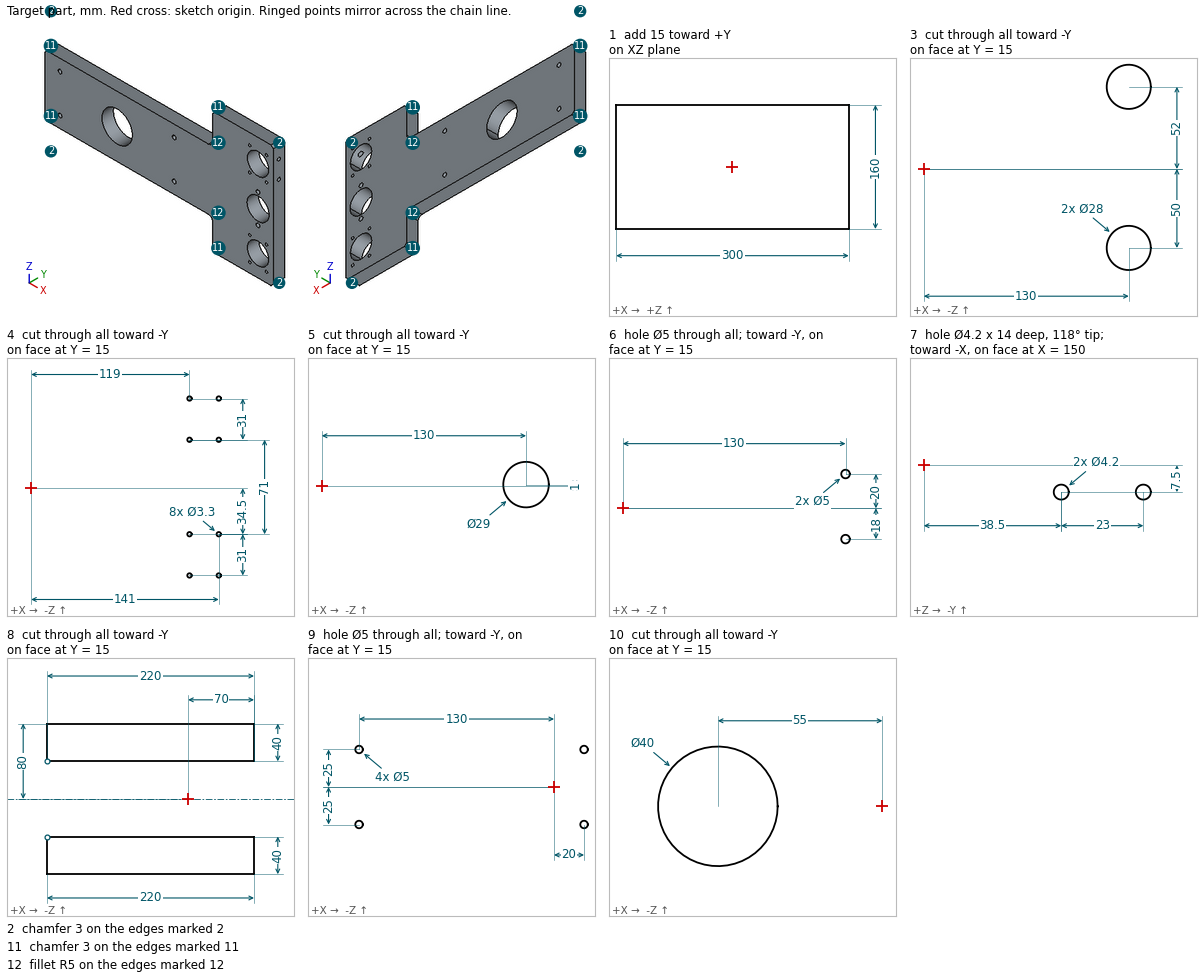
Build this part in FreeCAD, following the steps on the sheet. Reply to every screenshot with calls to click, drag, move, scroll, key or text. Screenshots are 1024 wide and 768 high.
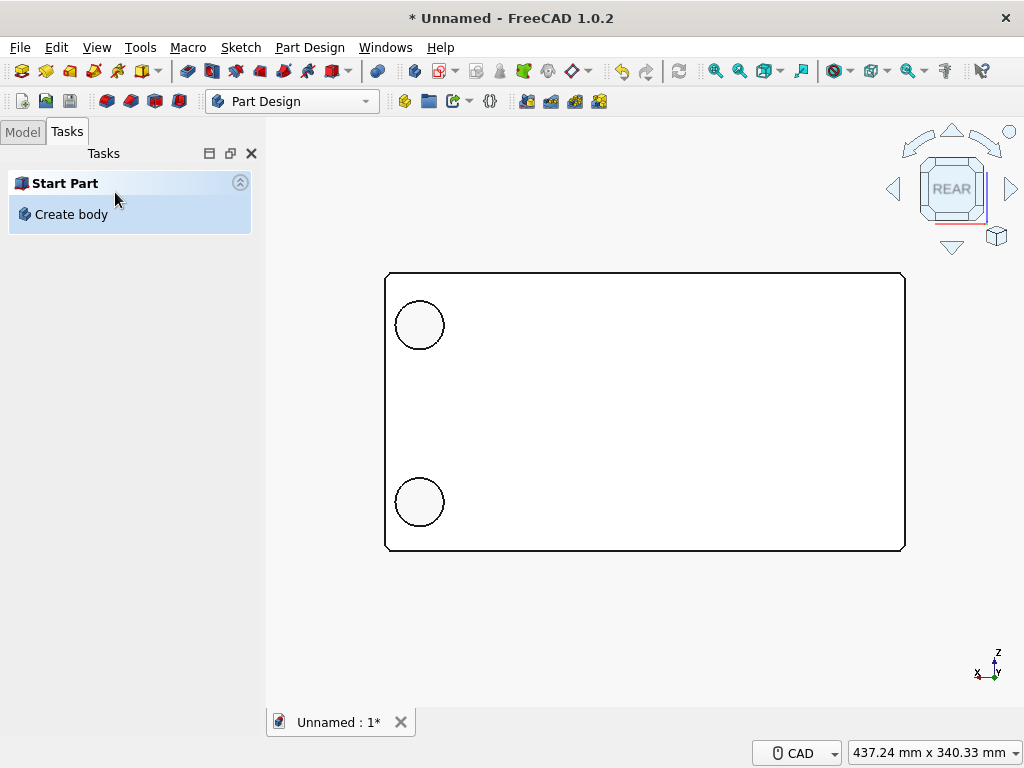
click(571, 411)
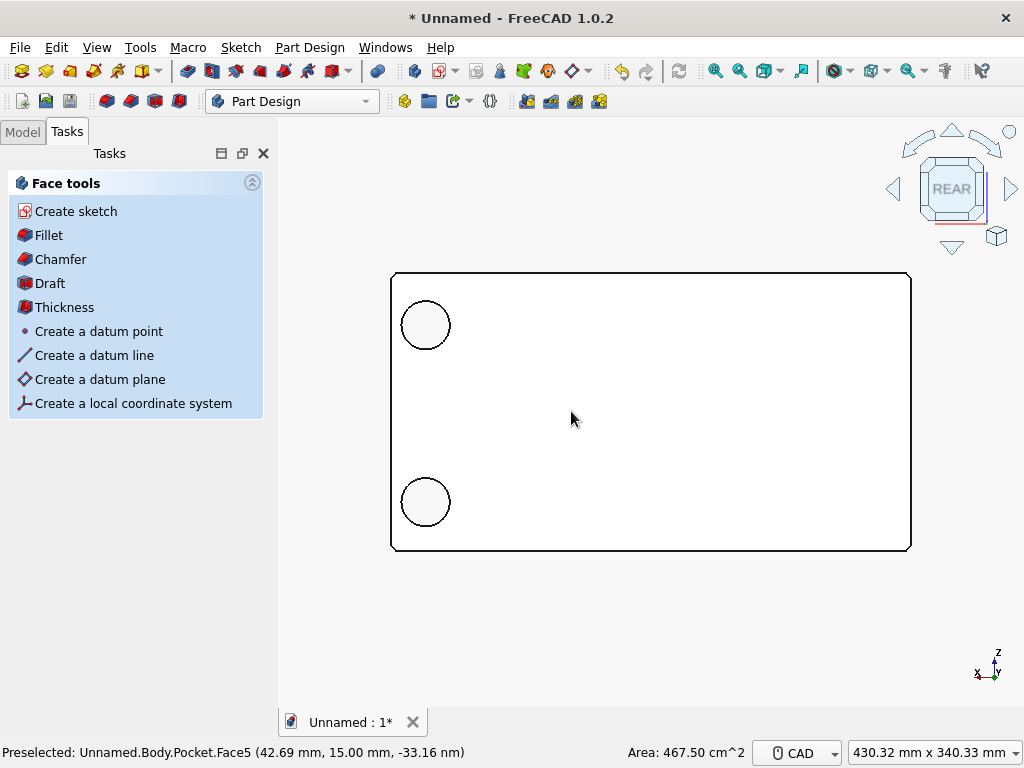
click(440, 72)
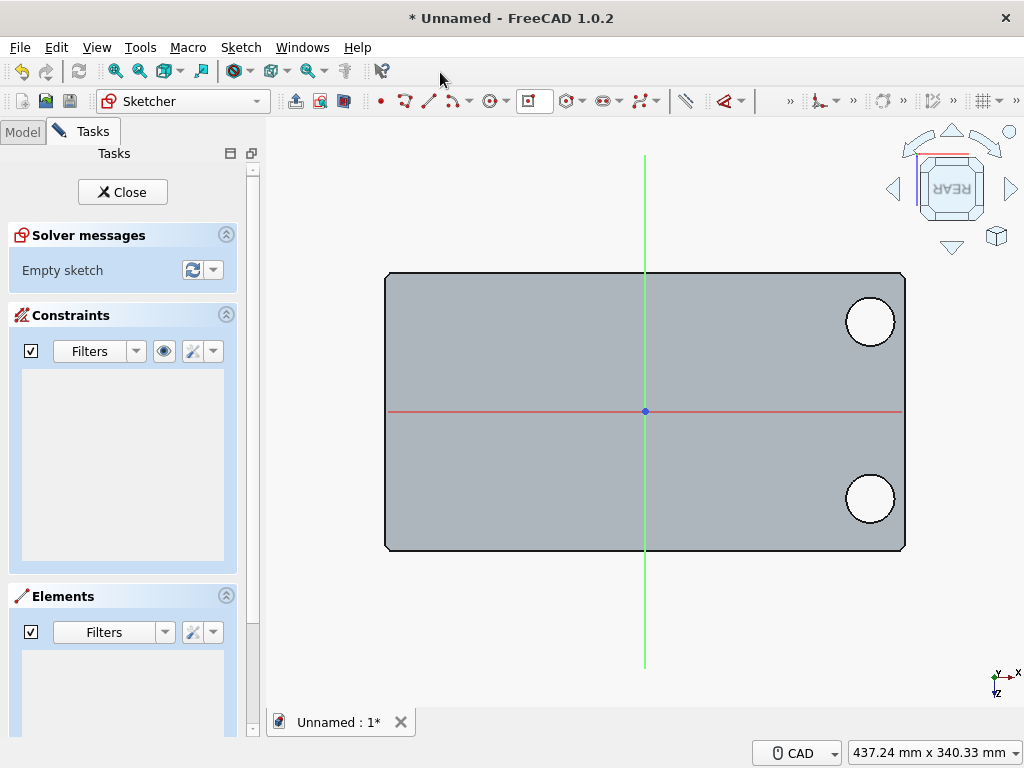
scroll(294, 420, down, 1)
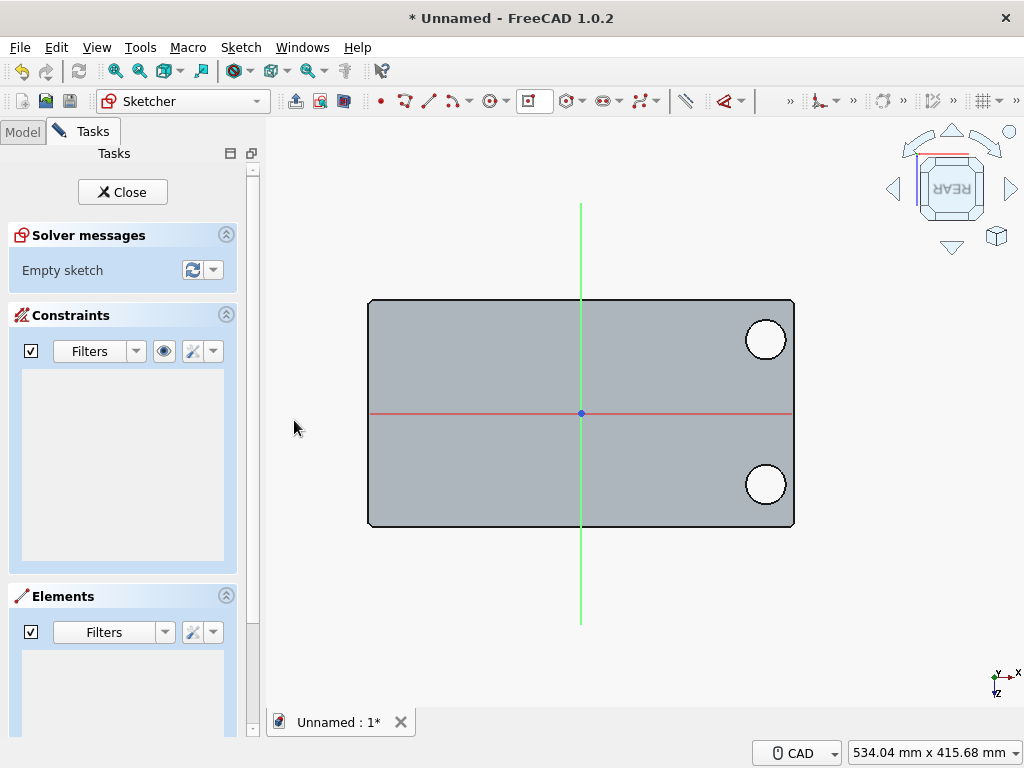
scroll(812, 412, up, 3)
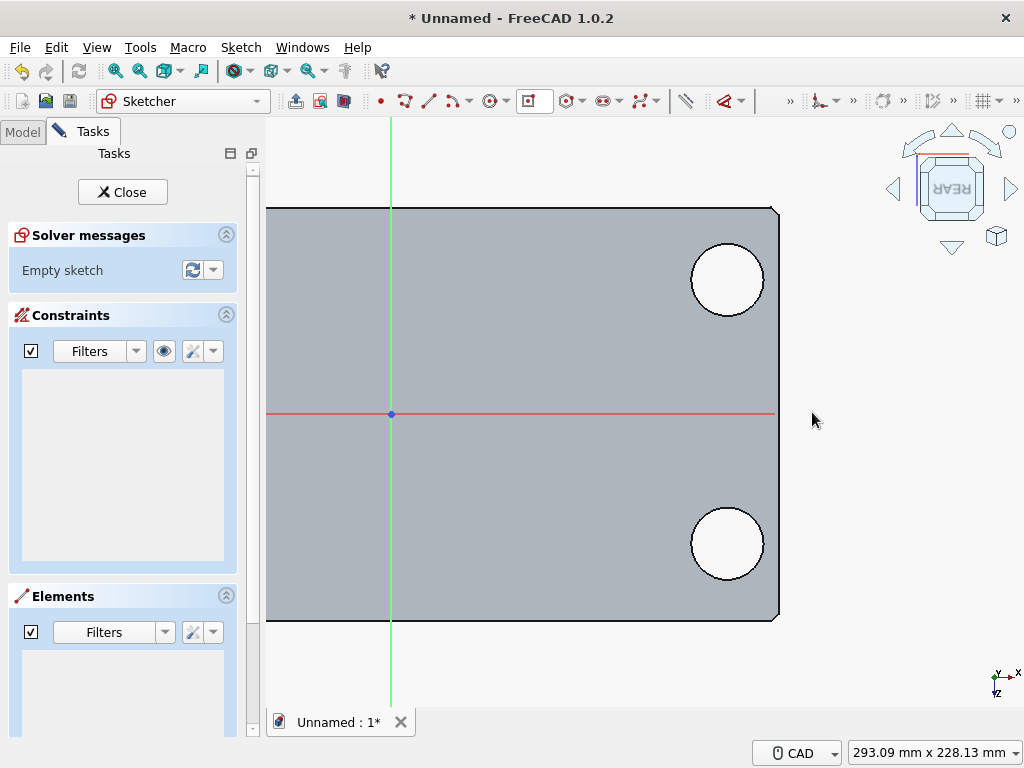
click(490, 102)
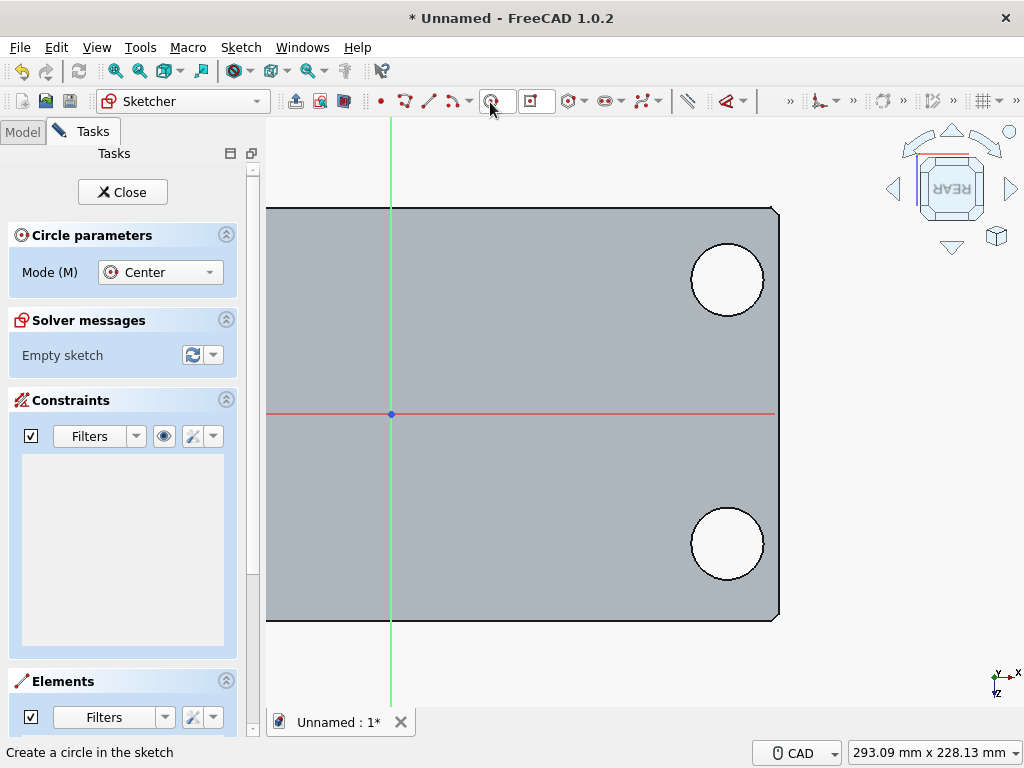
scroll(756, 504, up, 9)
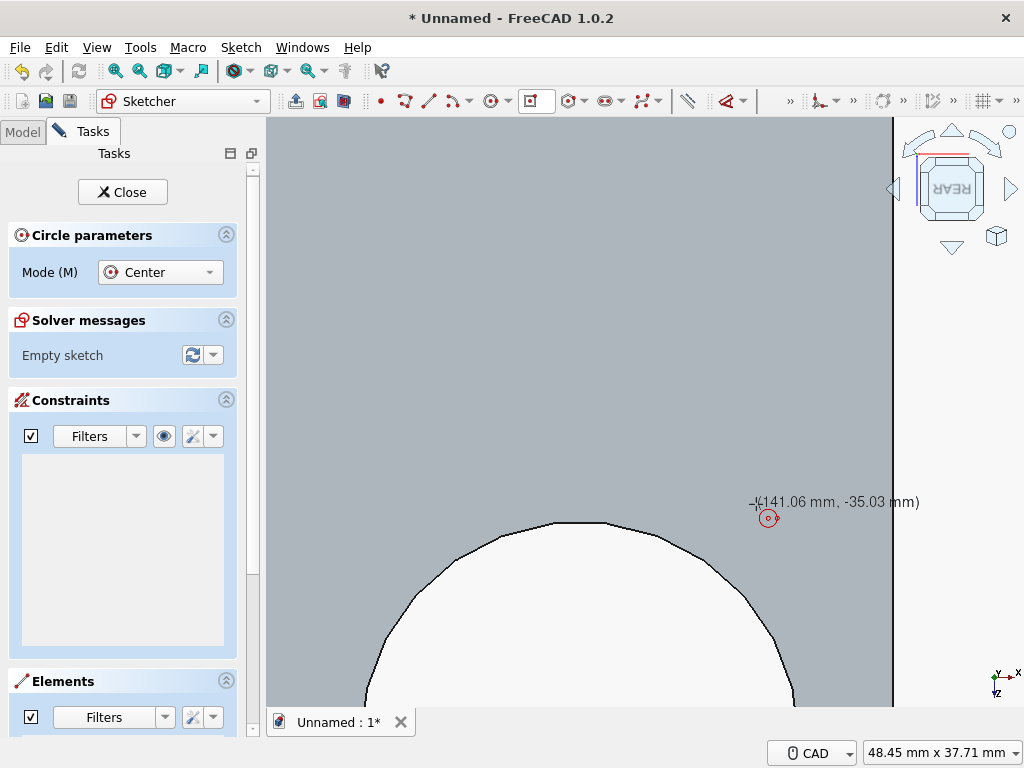
scroll(758, 505, down, 9)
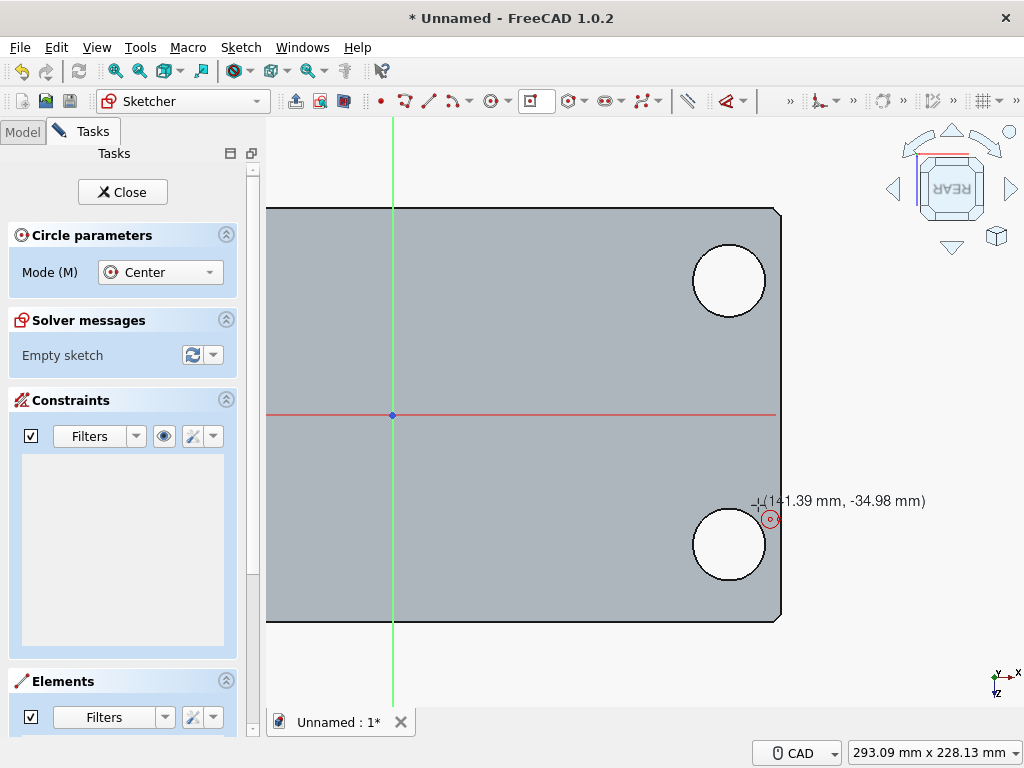
click(758, 504)
move(761, 501)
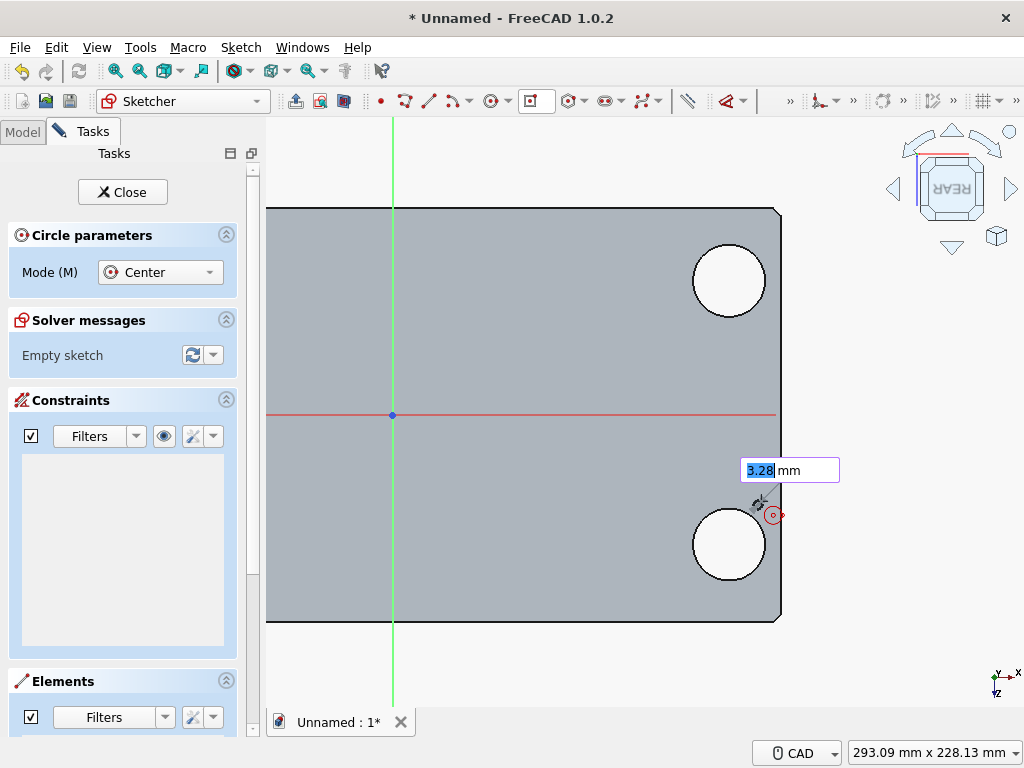
text(3.3)
key(Return)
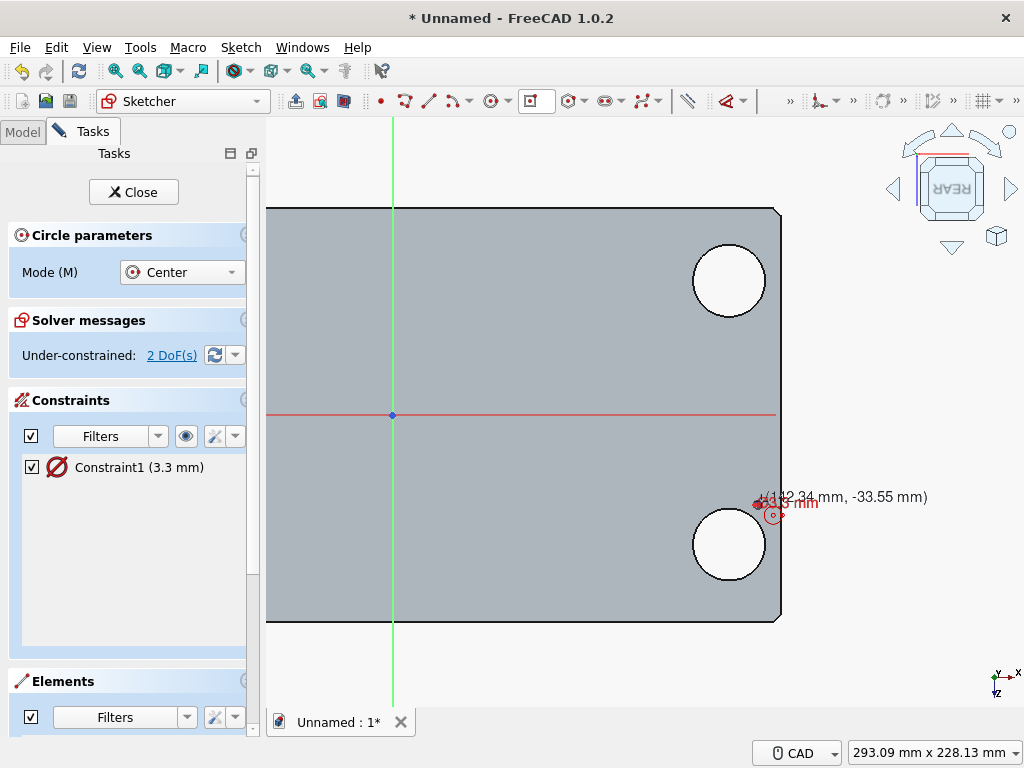
scroll(701, 241, up, 9)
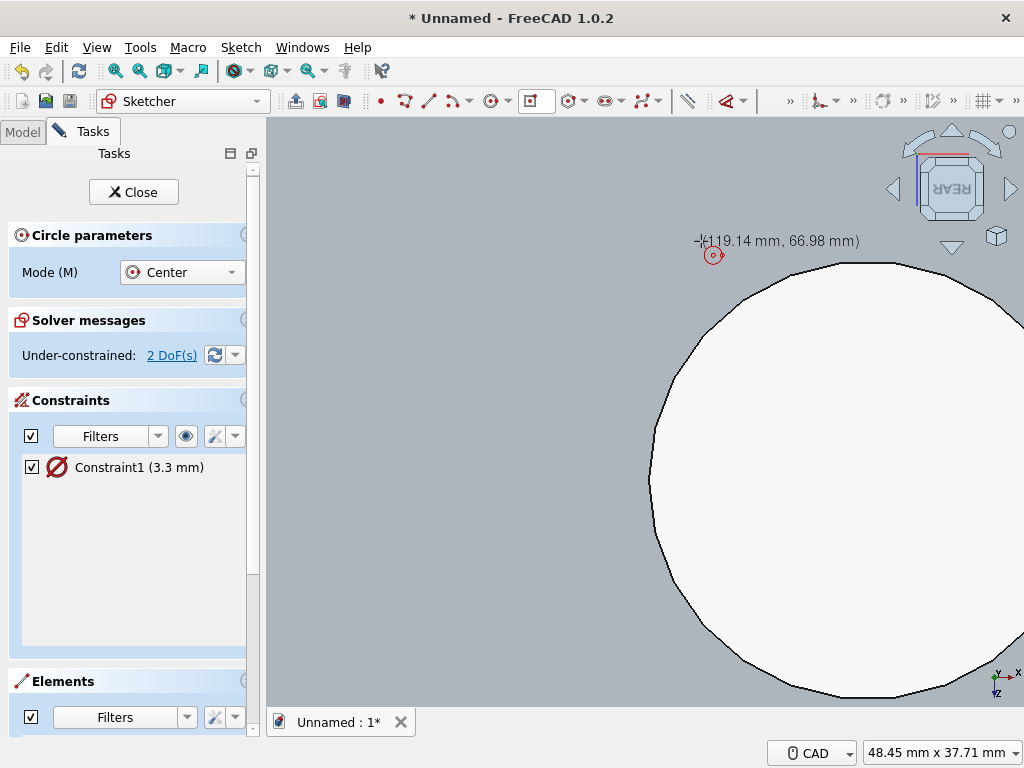
scroll(701, 240, down, 9)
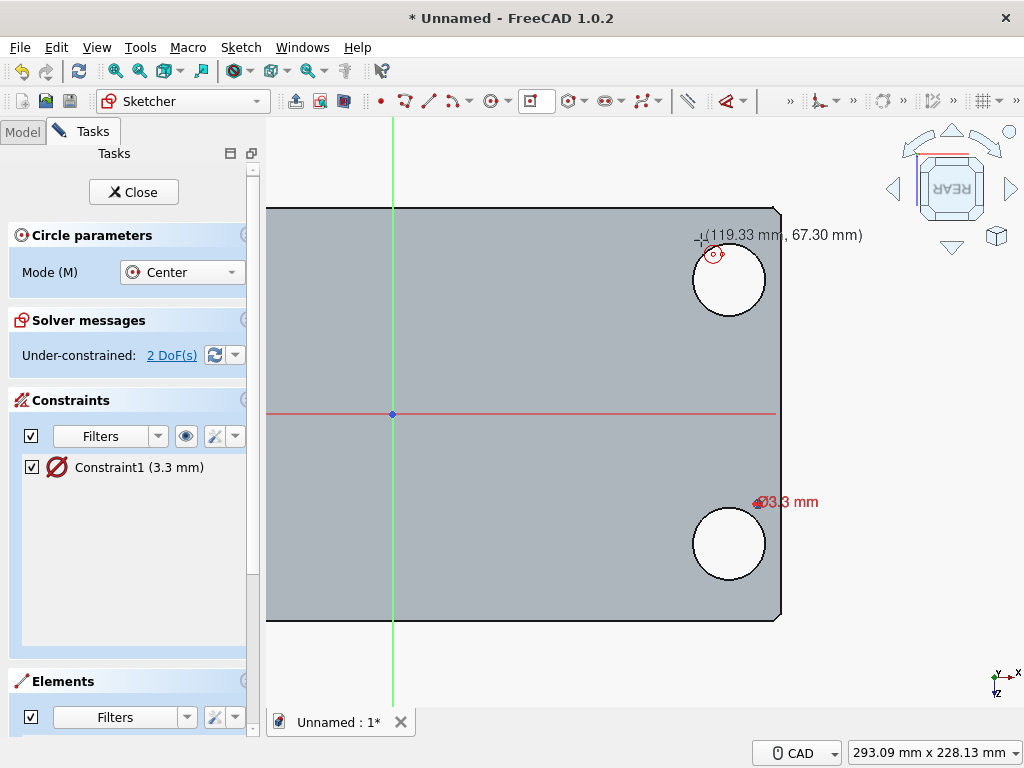
click(701, 240)
move(704, 237)